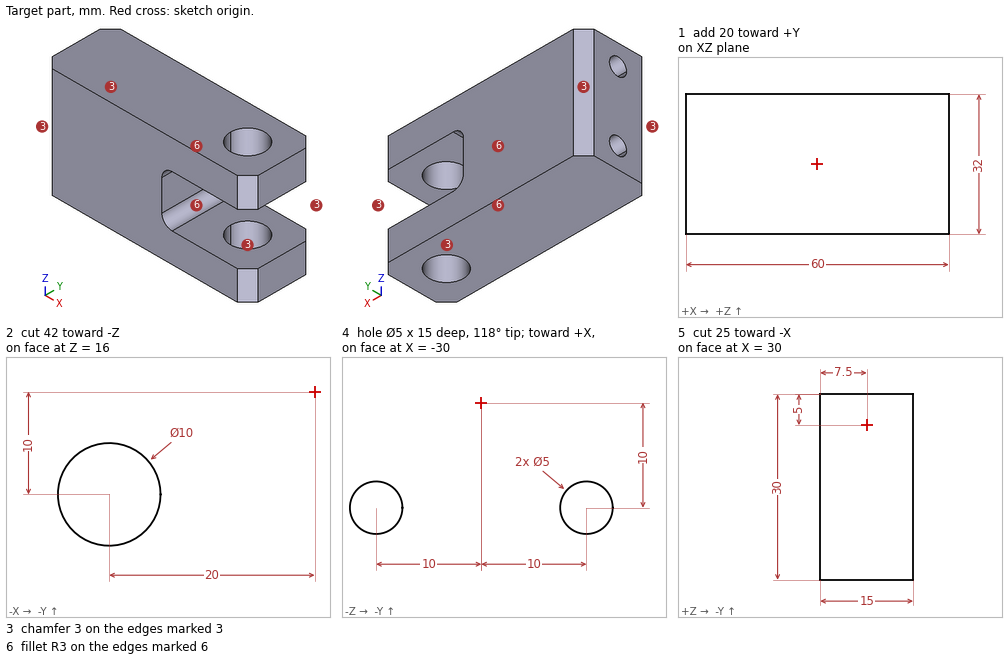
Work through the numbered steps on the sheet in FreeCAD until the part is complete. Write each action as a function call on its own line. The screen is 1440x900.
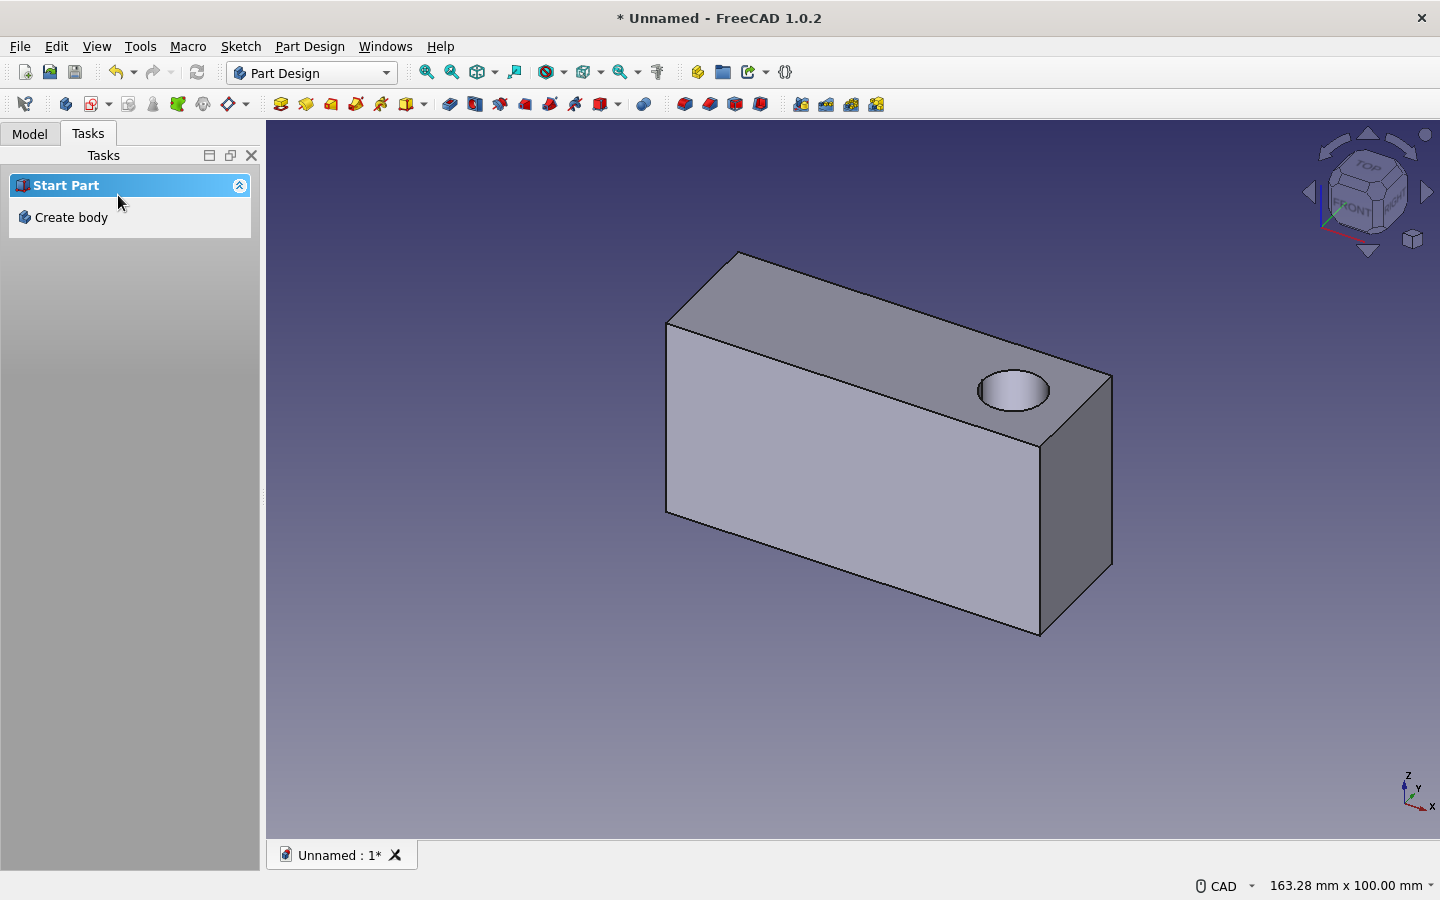
click(1040, 540)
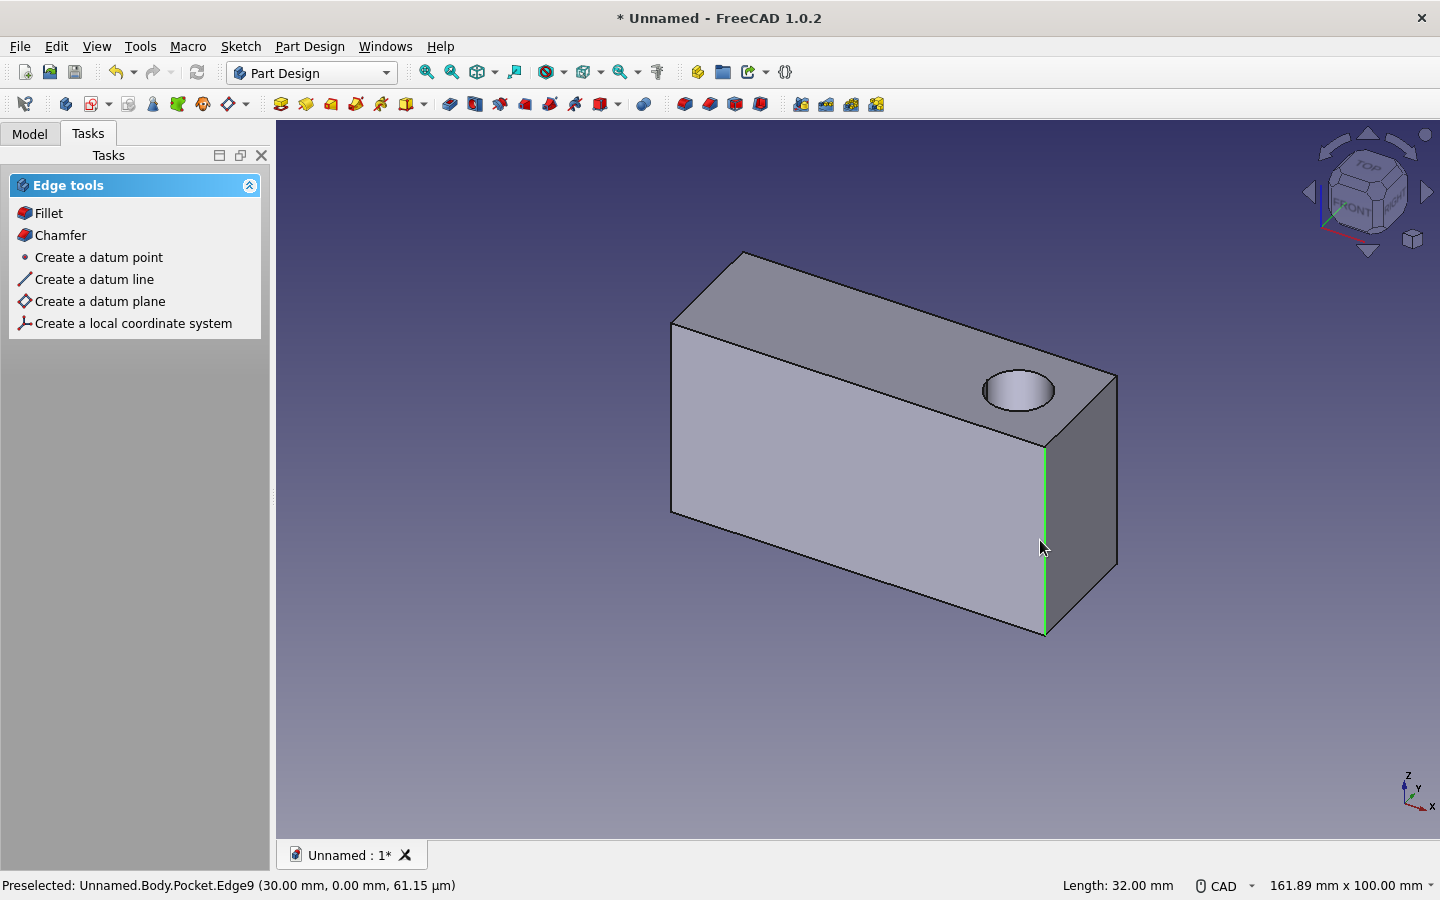
key(0)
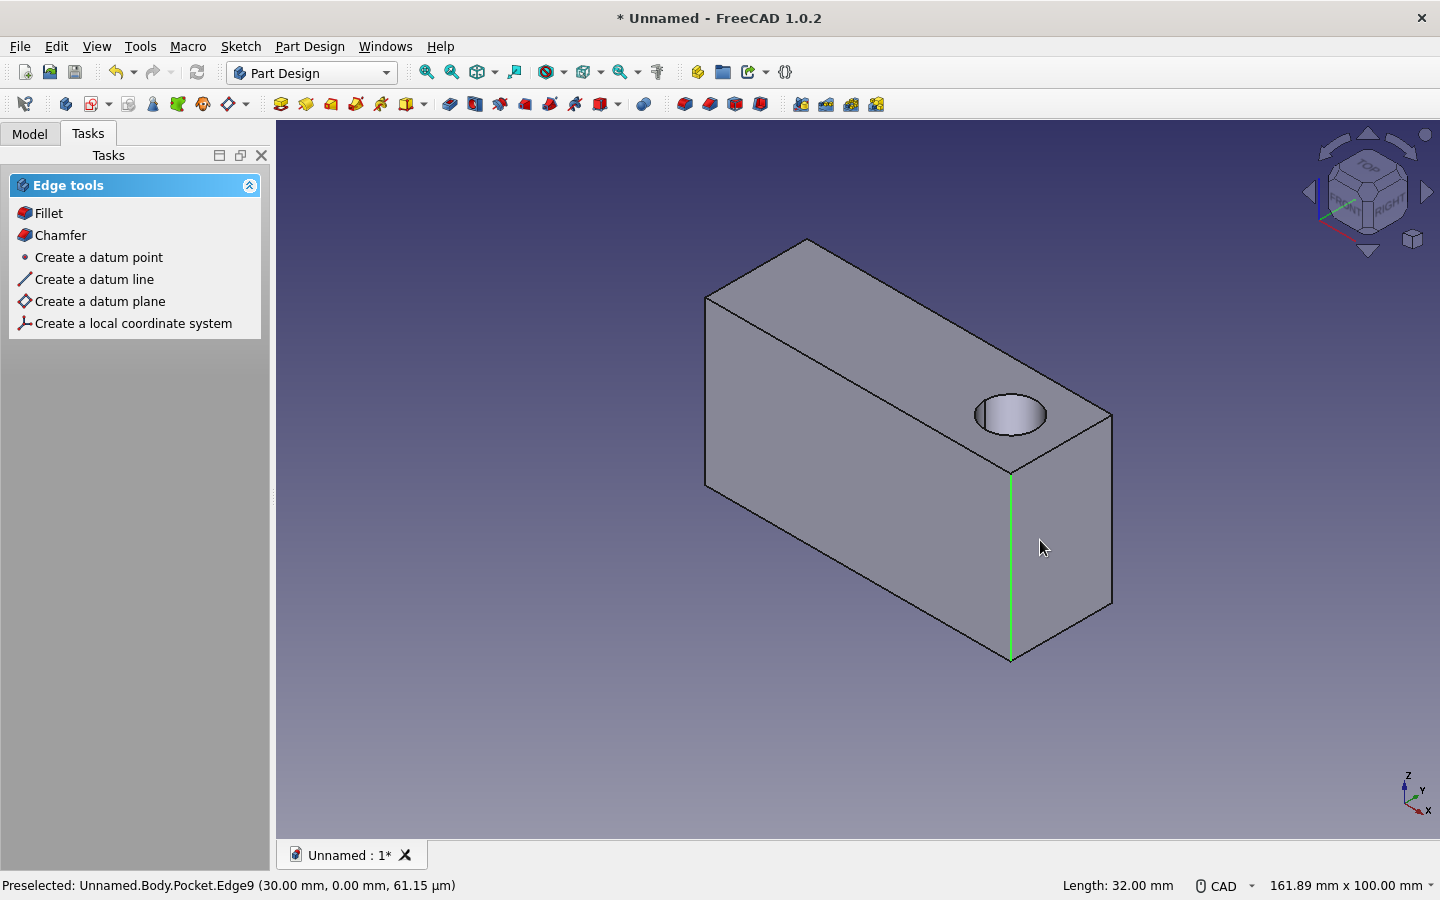
key(2)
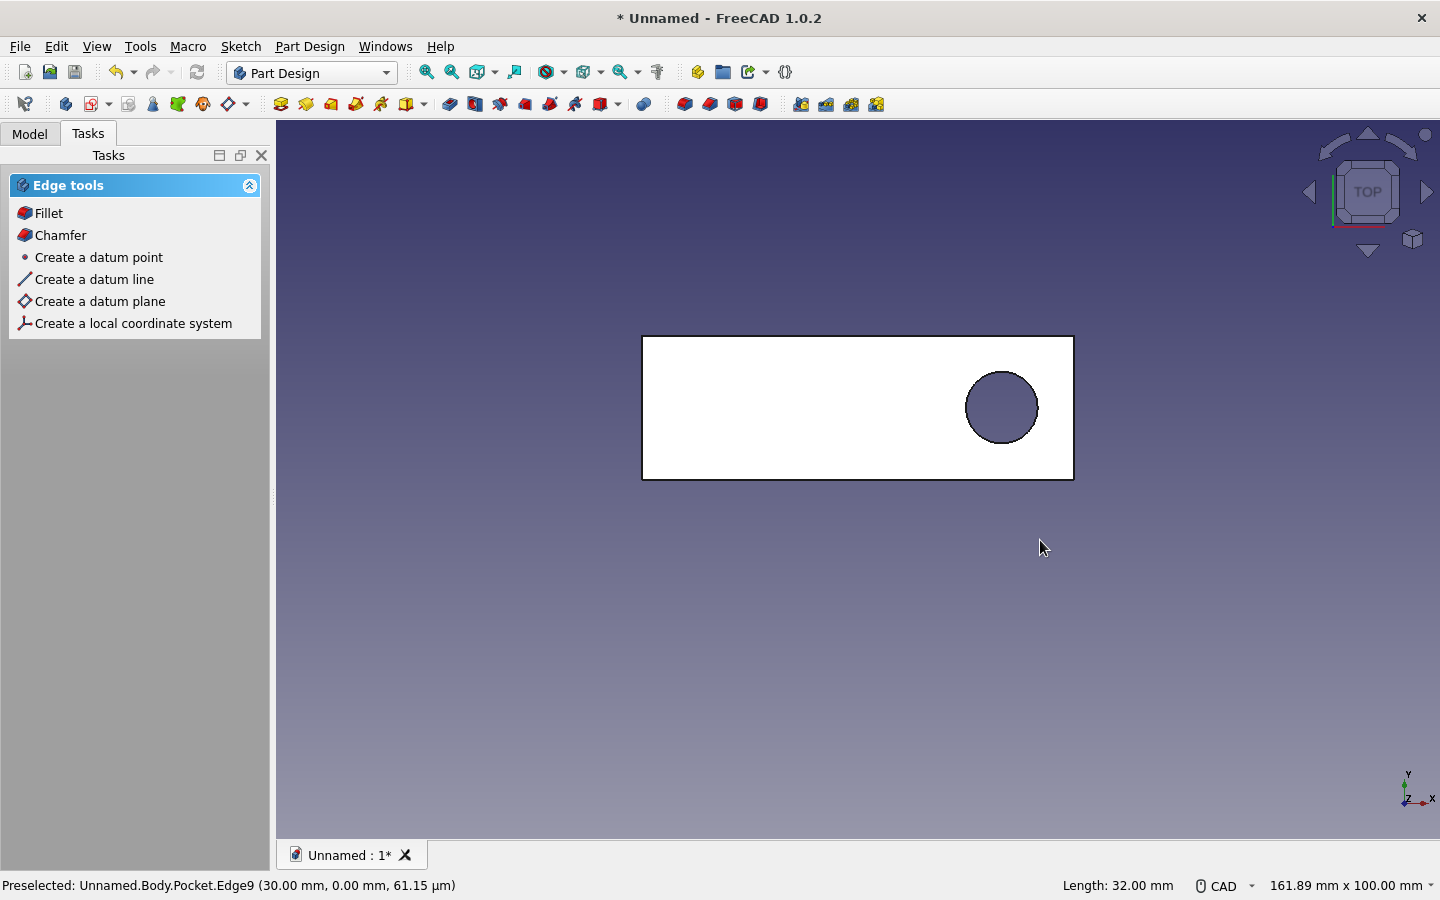
click(427, 72)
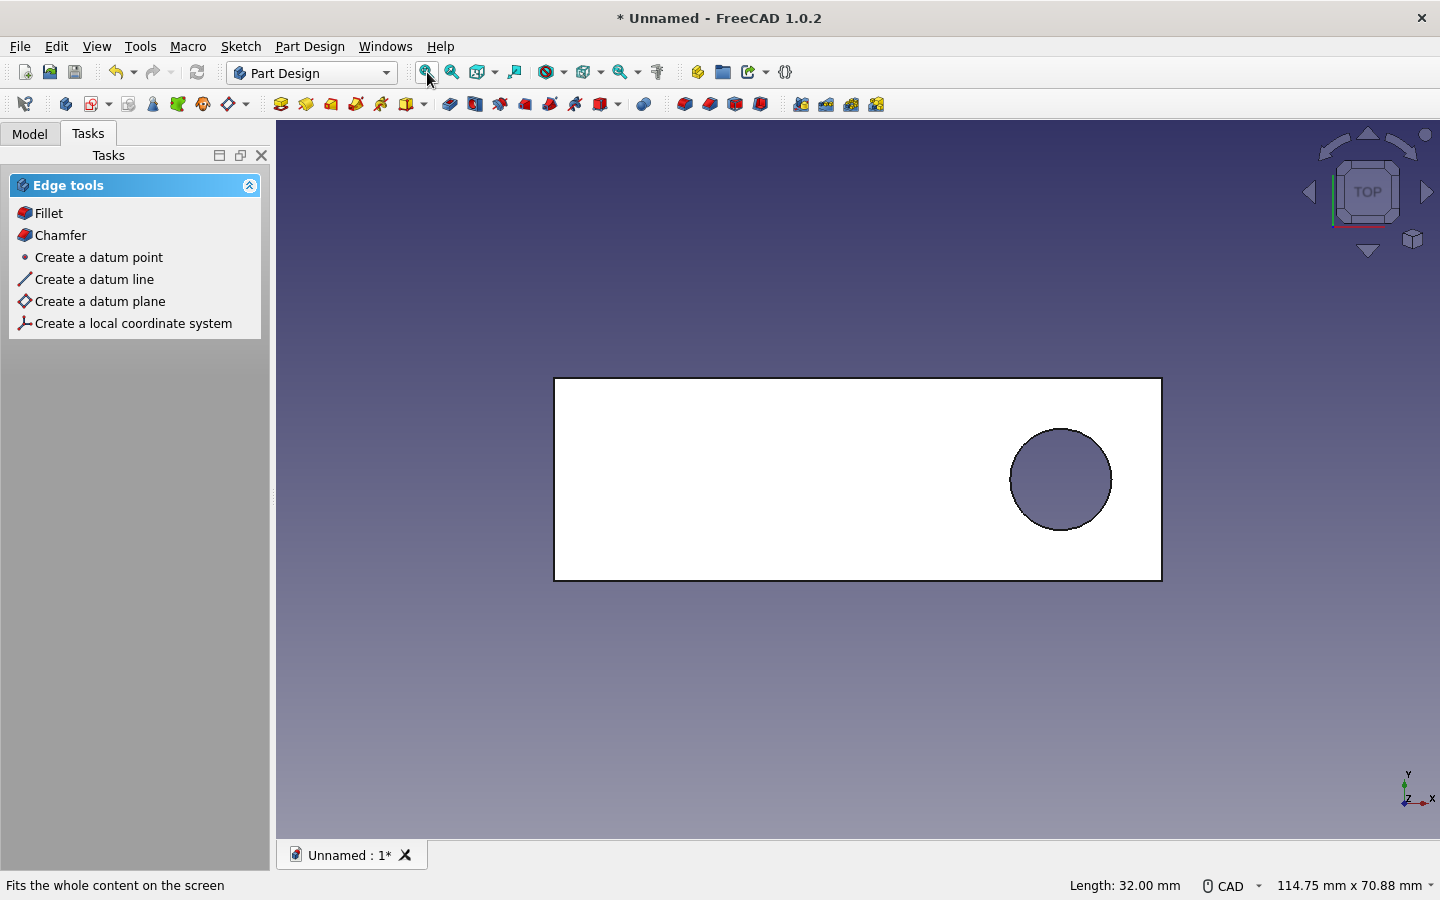
key(1)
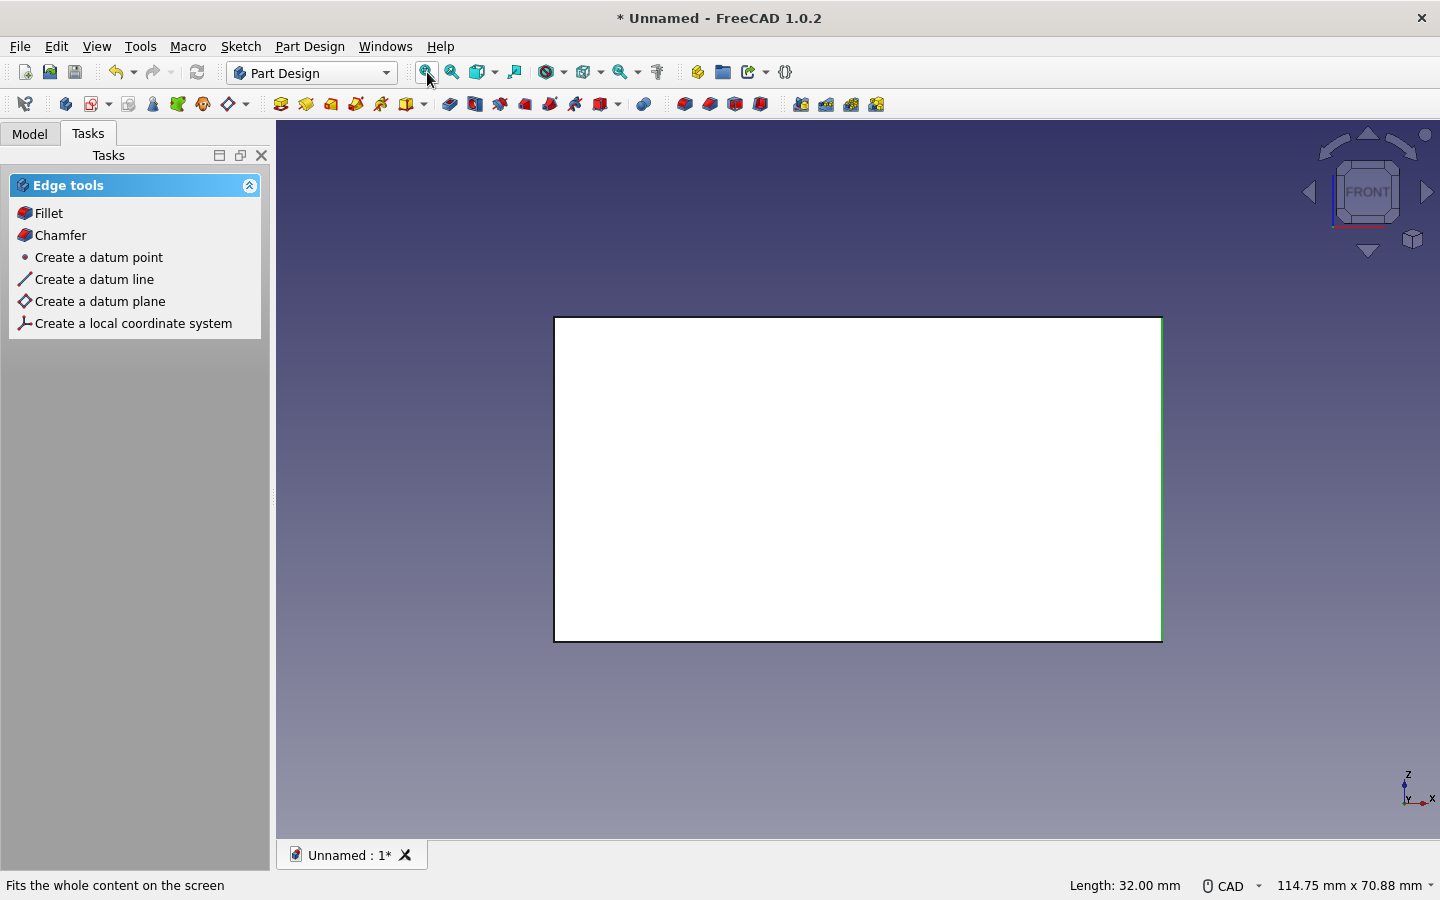
click(554, 446, ctrl)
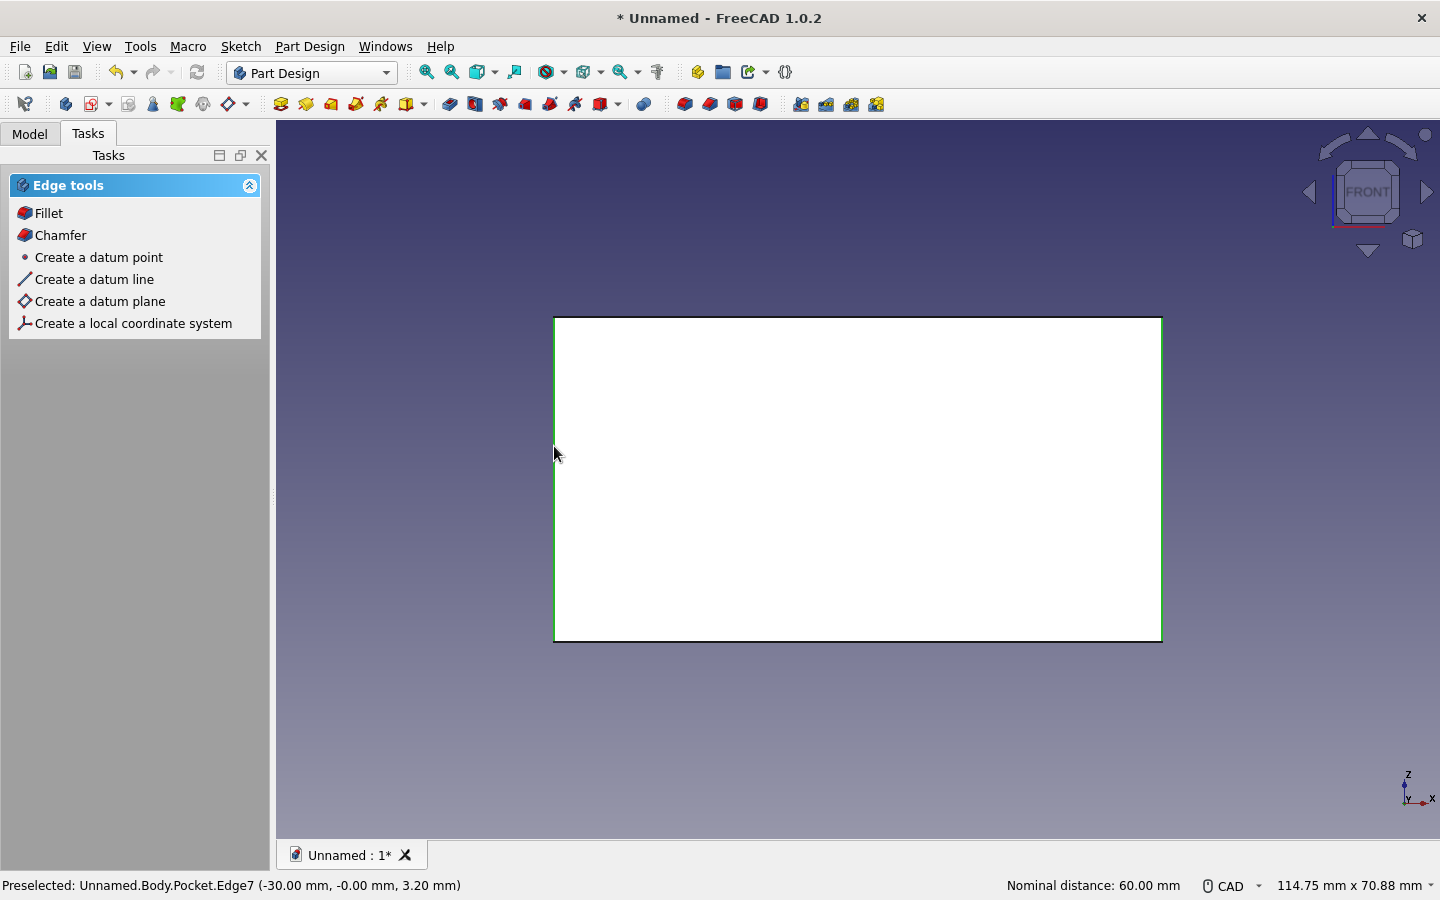
key(3)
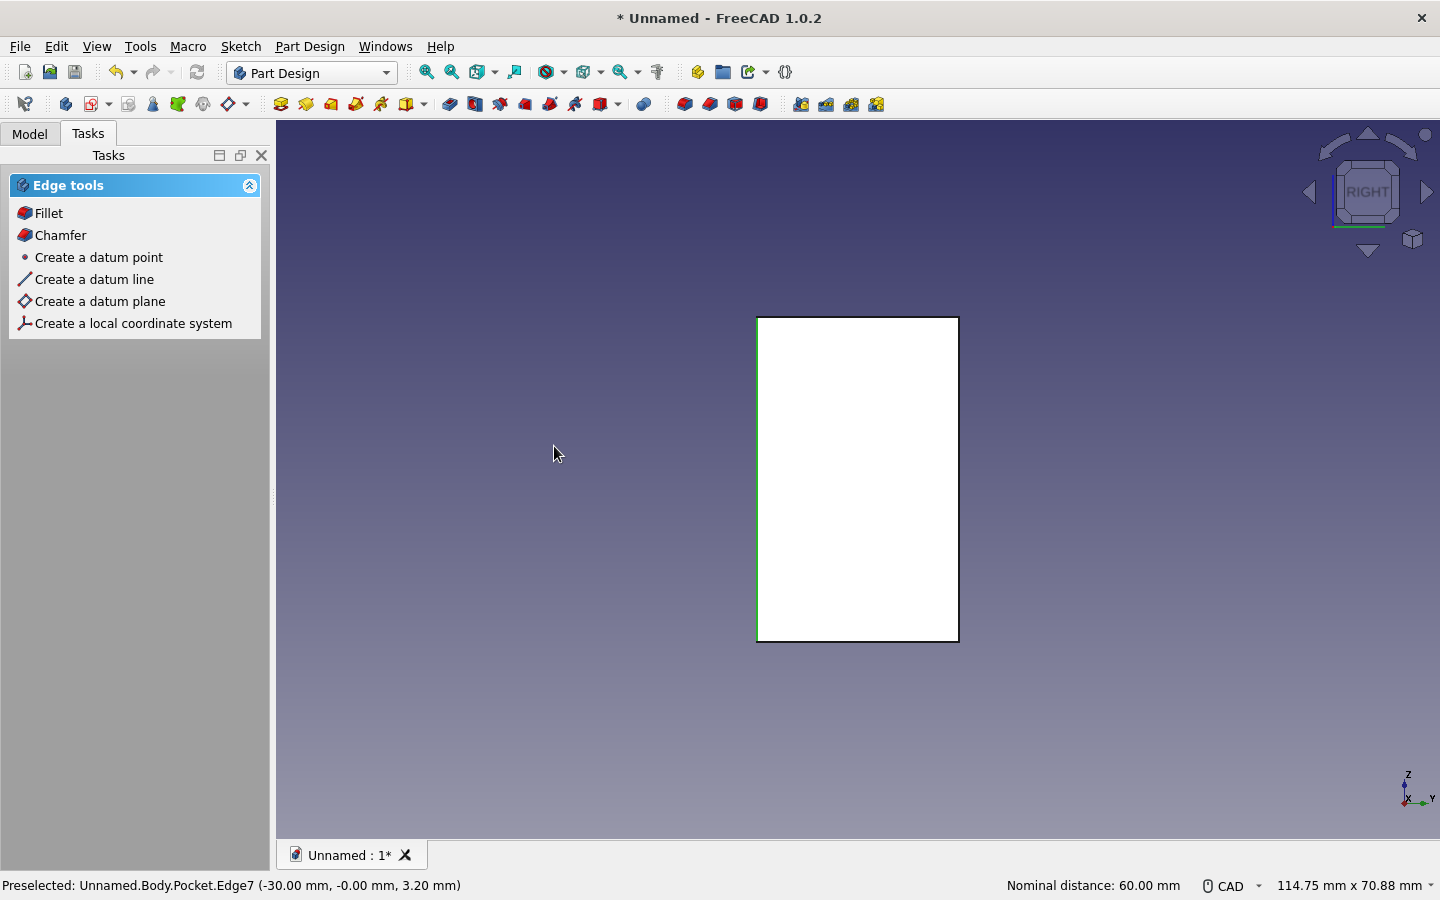
click(959, 478, ctrl)